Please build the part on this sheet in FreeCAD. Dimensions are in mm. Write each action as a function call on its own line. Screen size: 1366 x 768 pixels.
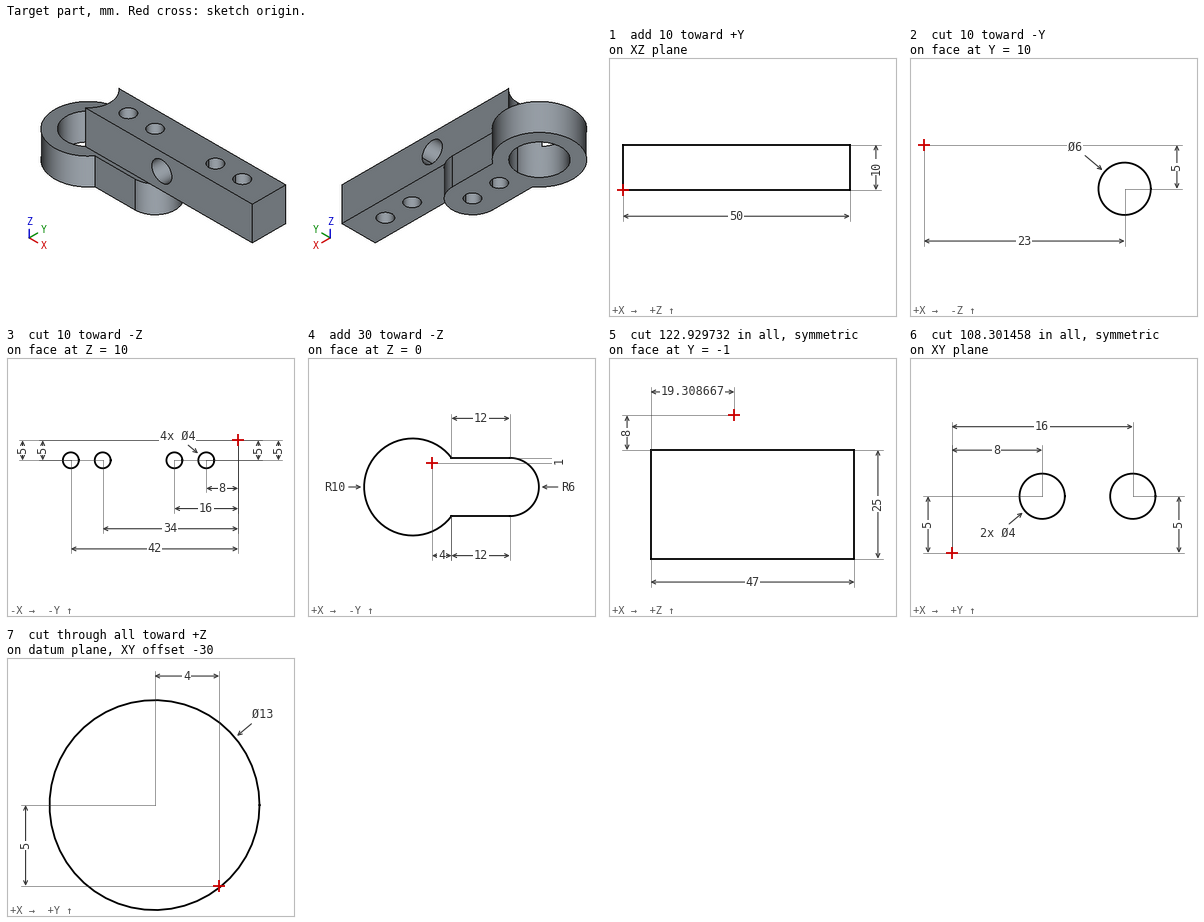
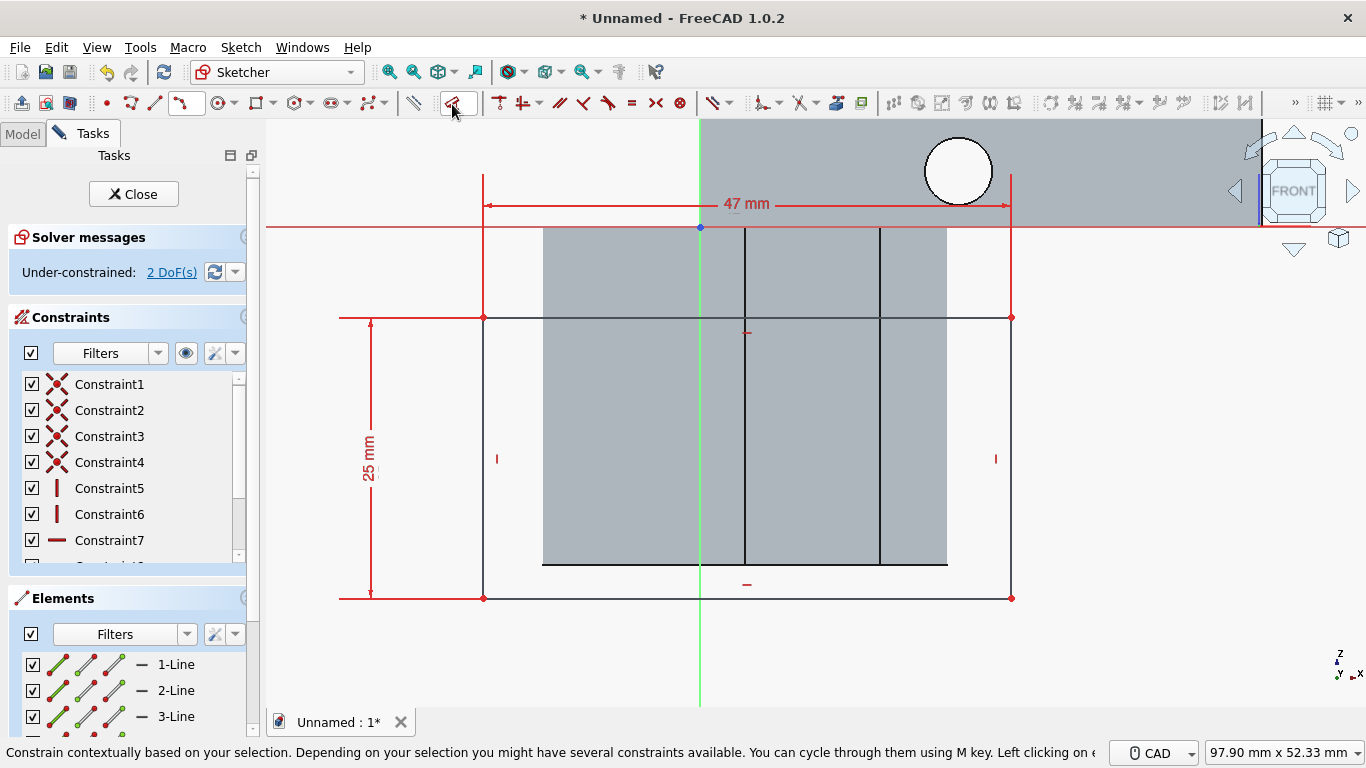
click(483, 318)
click(449, 273)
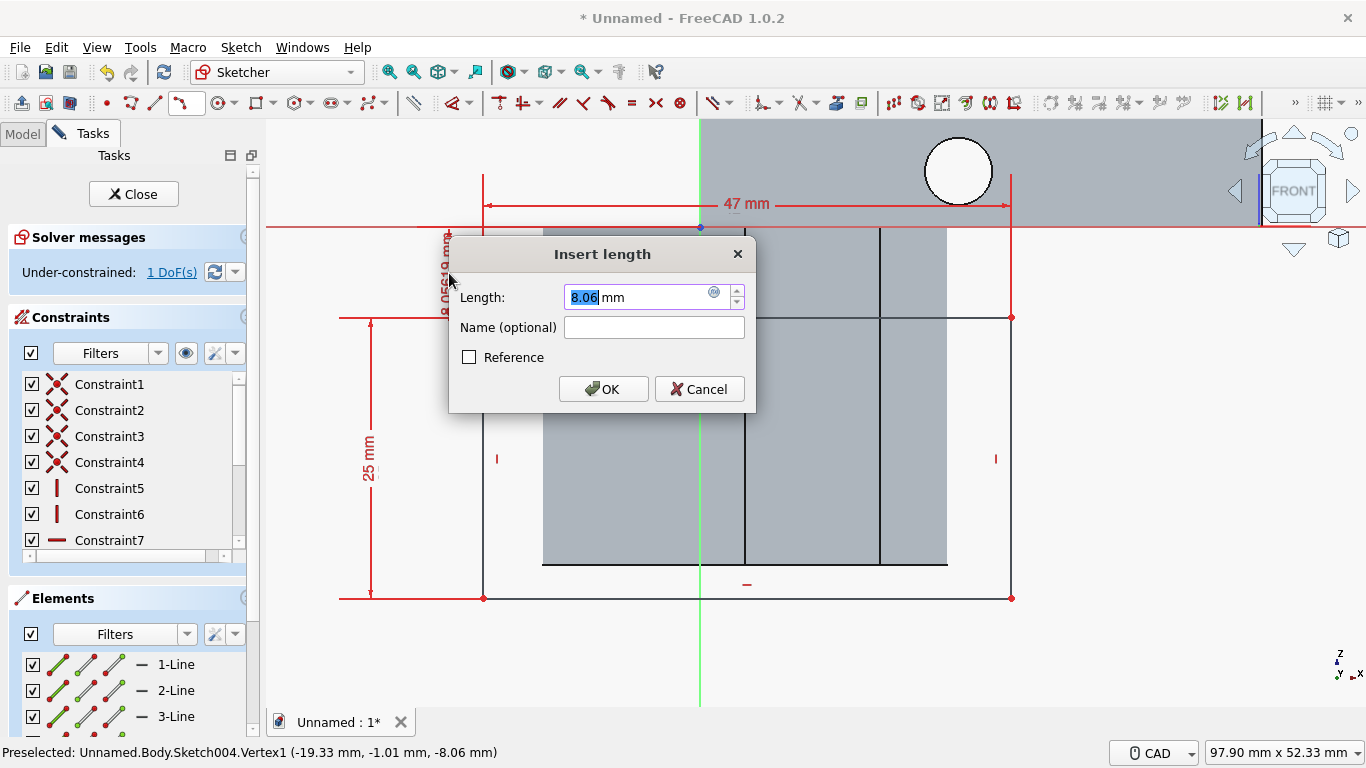
text(8)
key(Return)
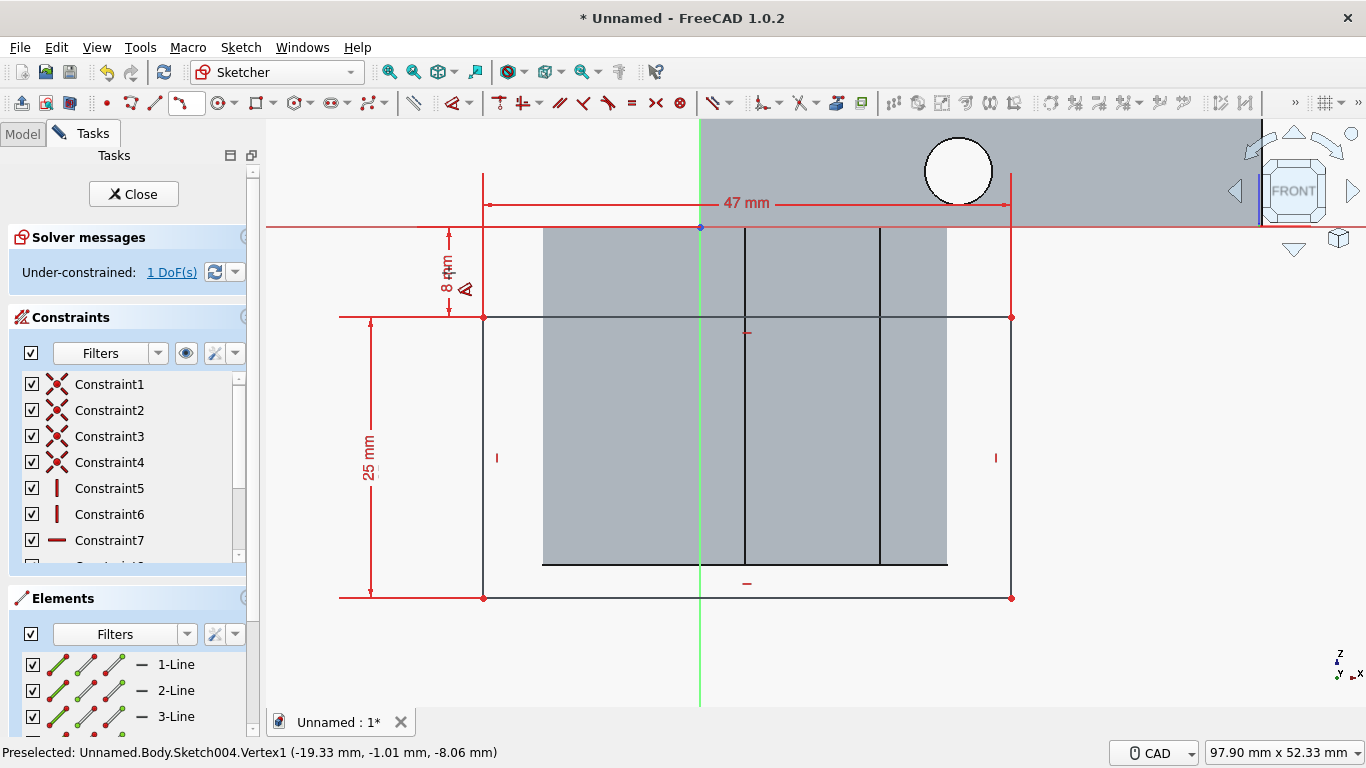
click(483, 317)
click(592, 193)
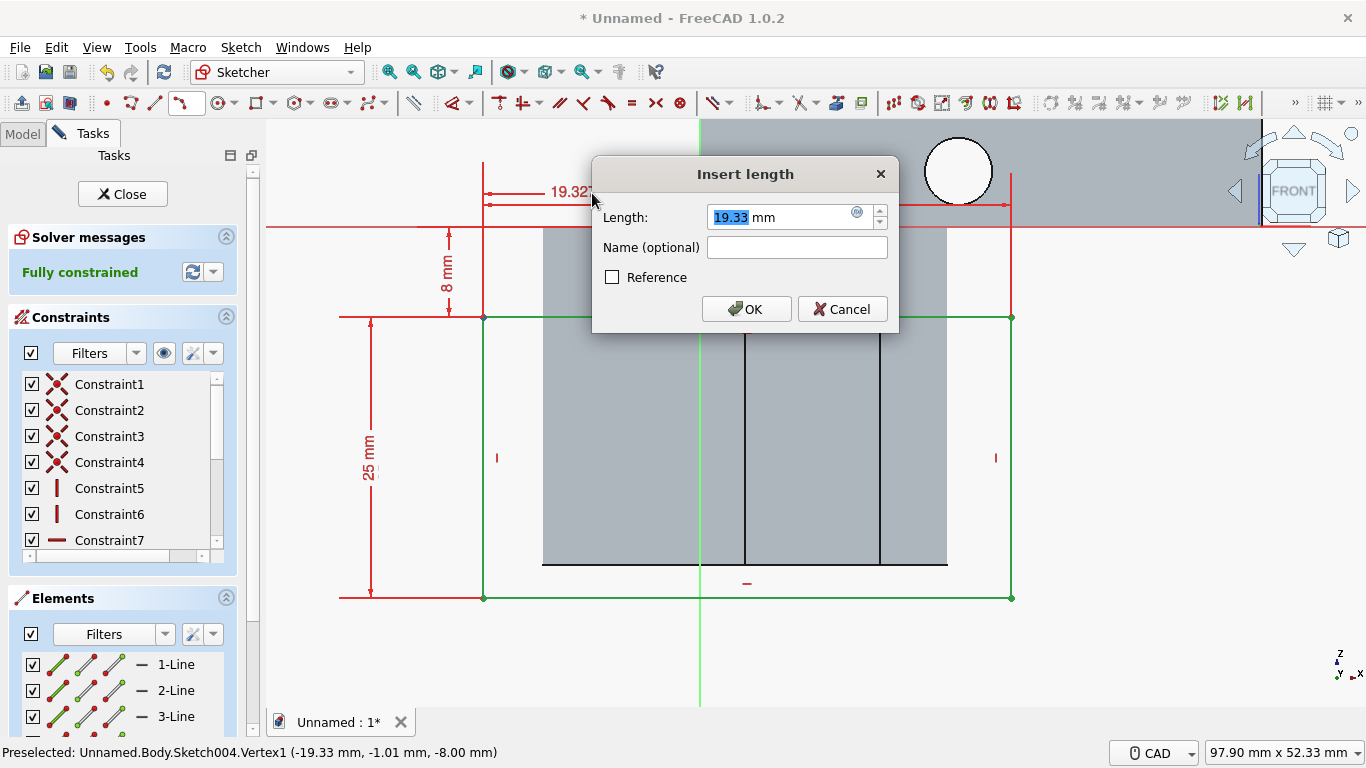
text(19.308667)
key(Return)
key(Escape)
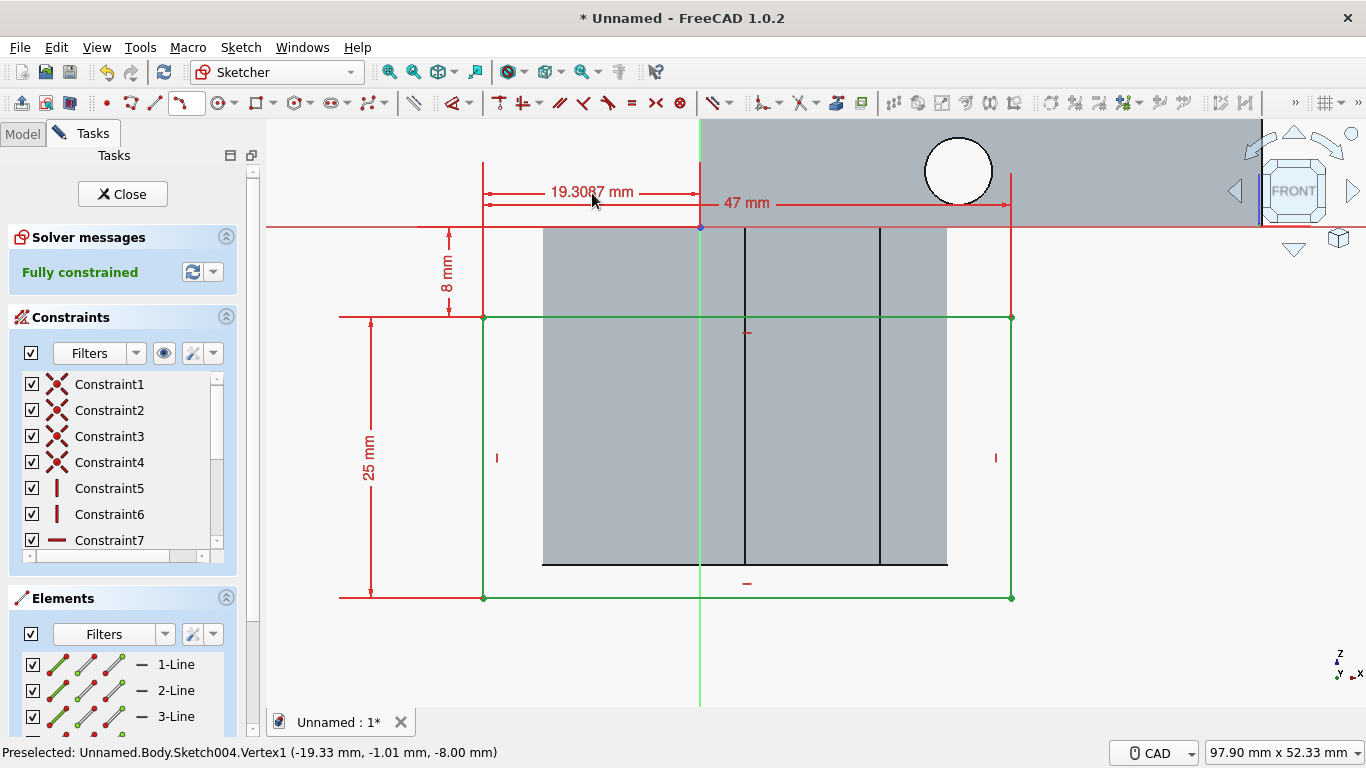
click(123, 194)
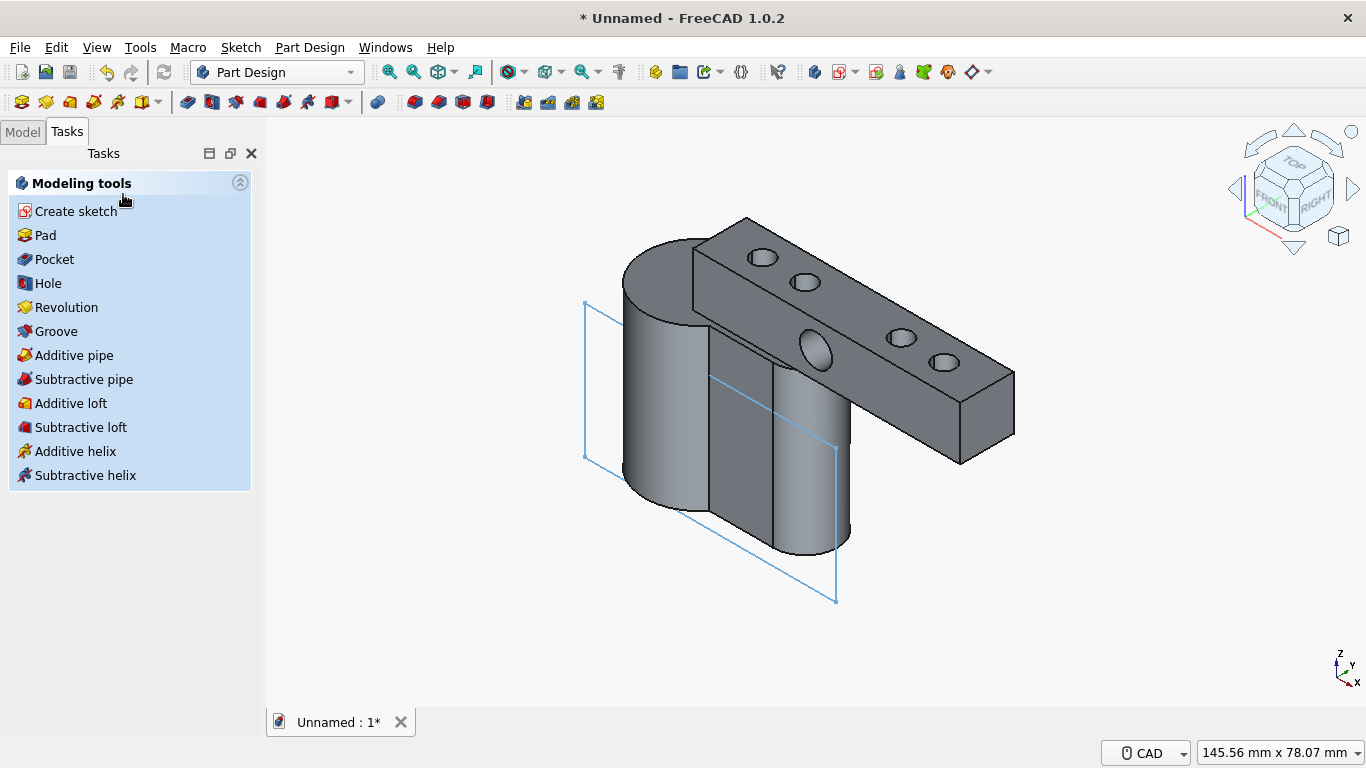
click(188, 102)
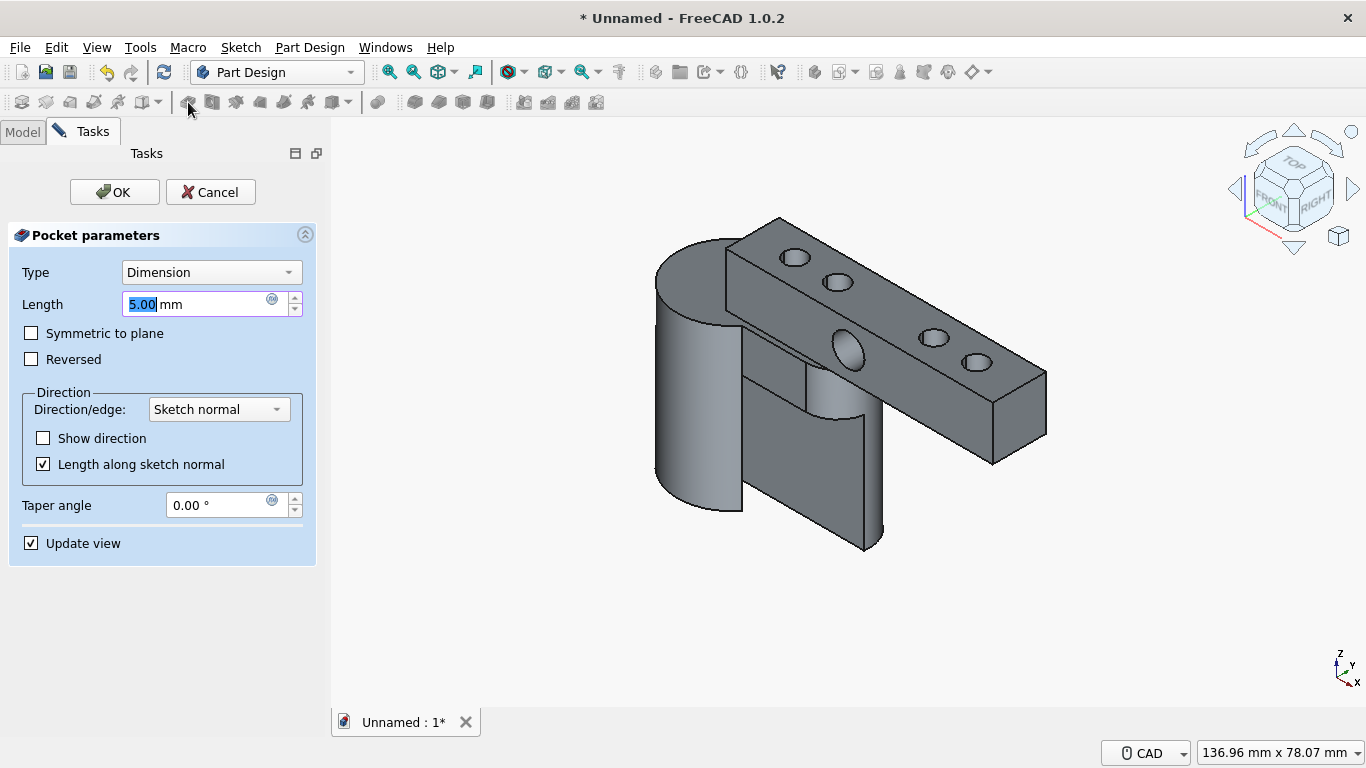
text(122.929732)
key(Tab)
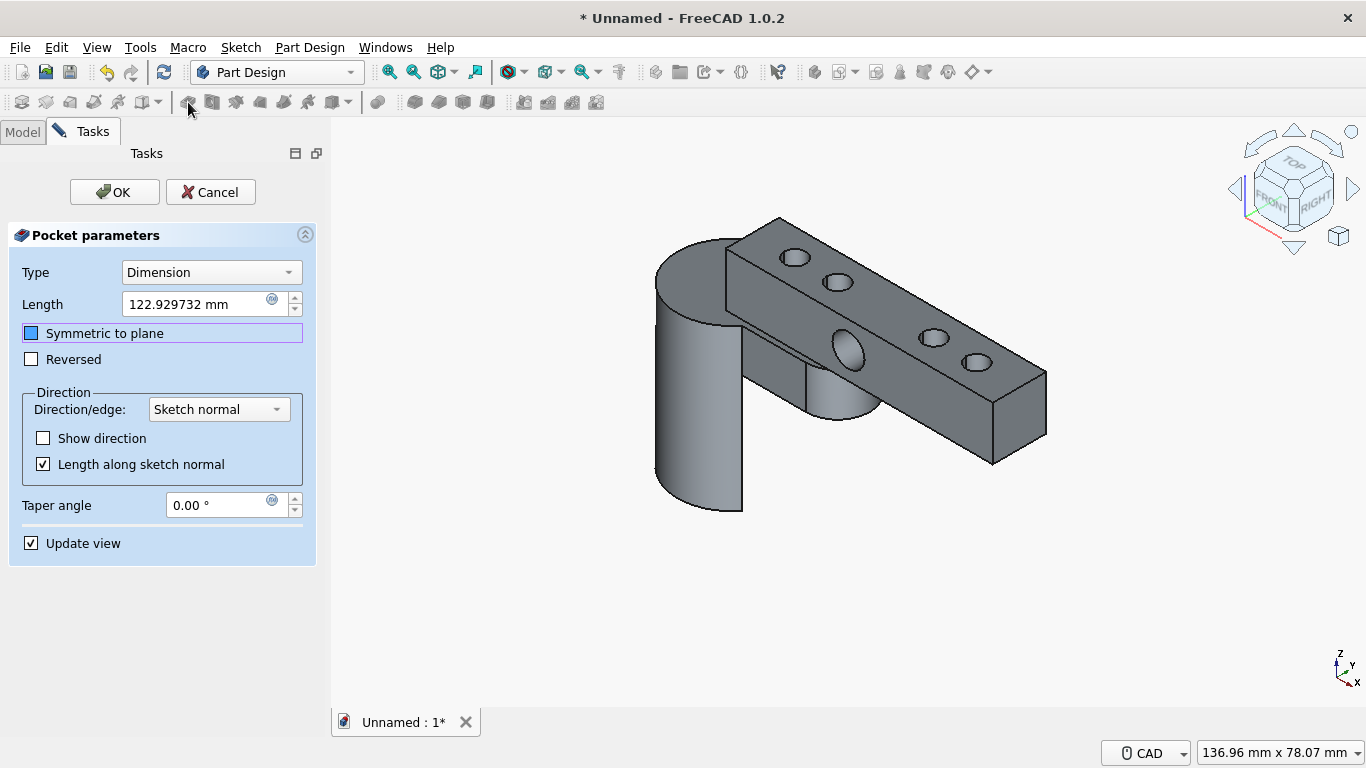
click(30, 333)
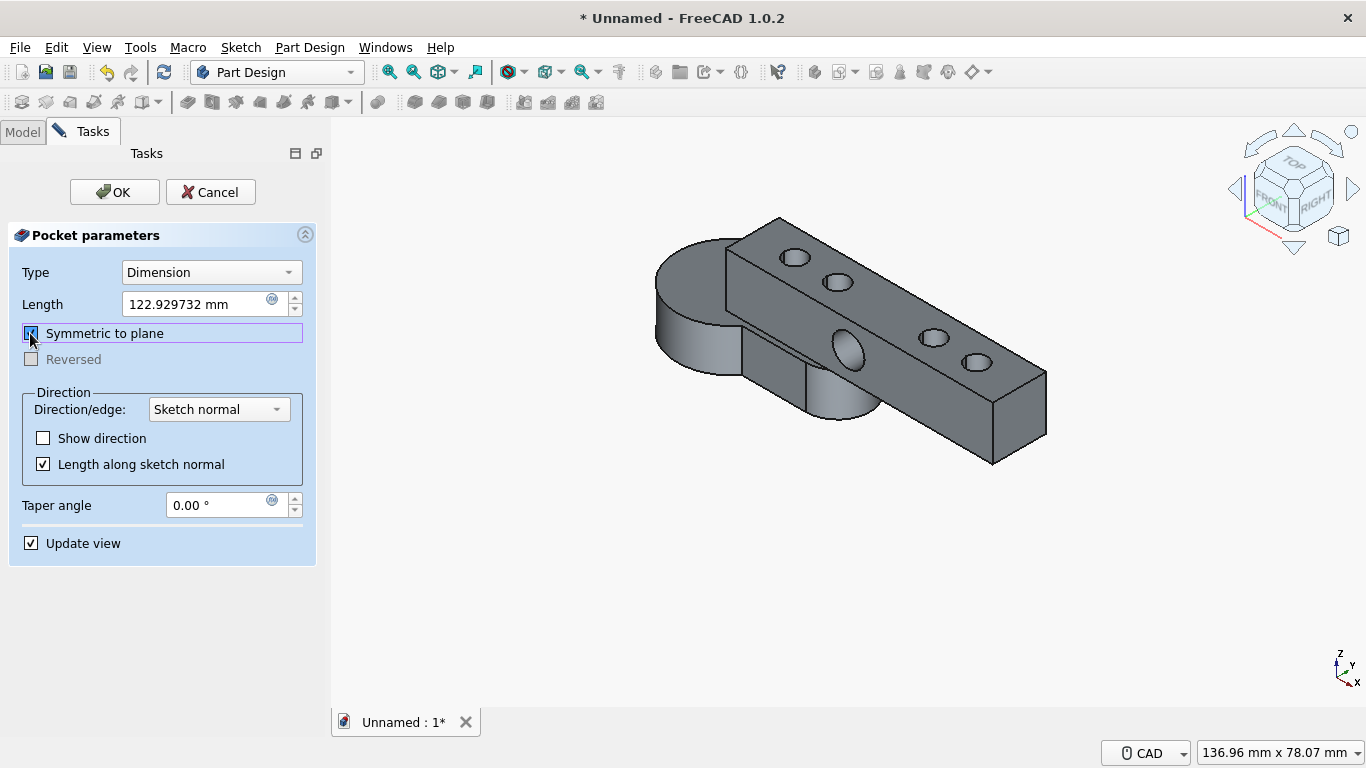
click(115, 192)